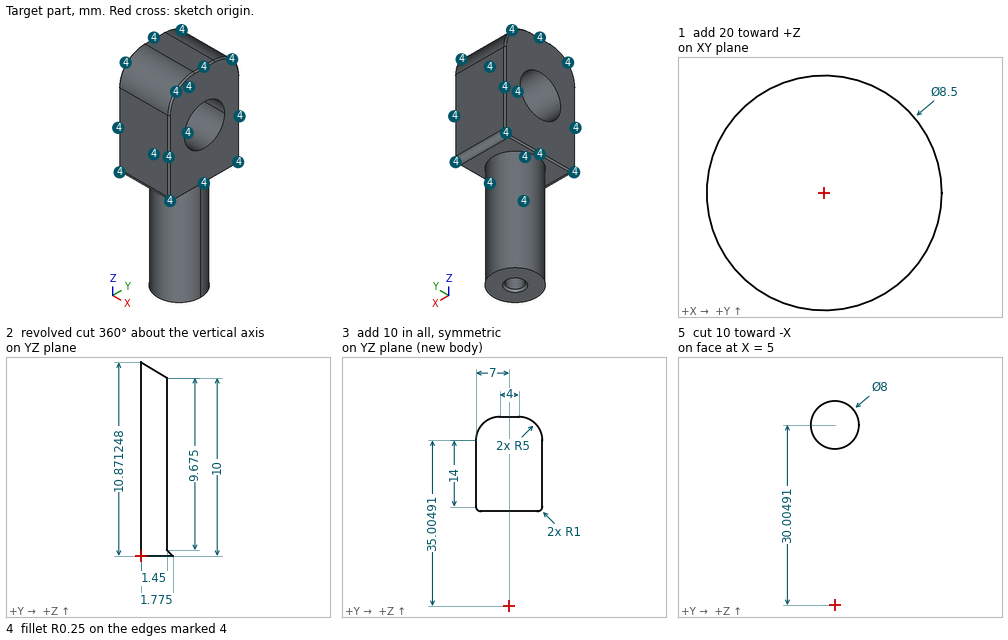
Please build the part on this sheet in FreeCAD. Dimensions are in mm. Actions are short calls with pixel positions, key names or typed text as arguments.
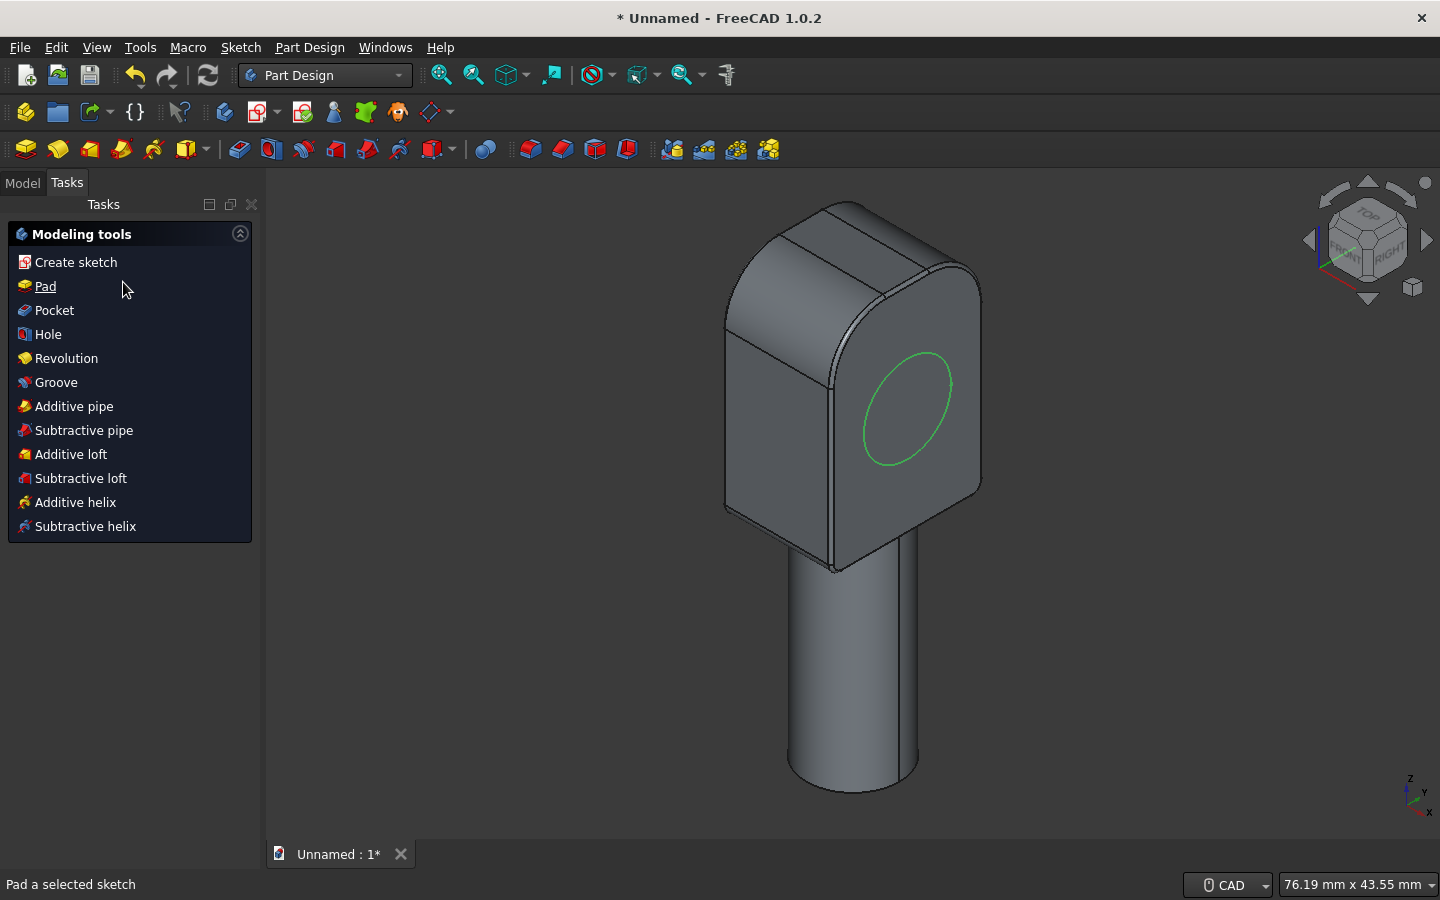
click(240, 150)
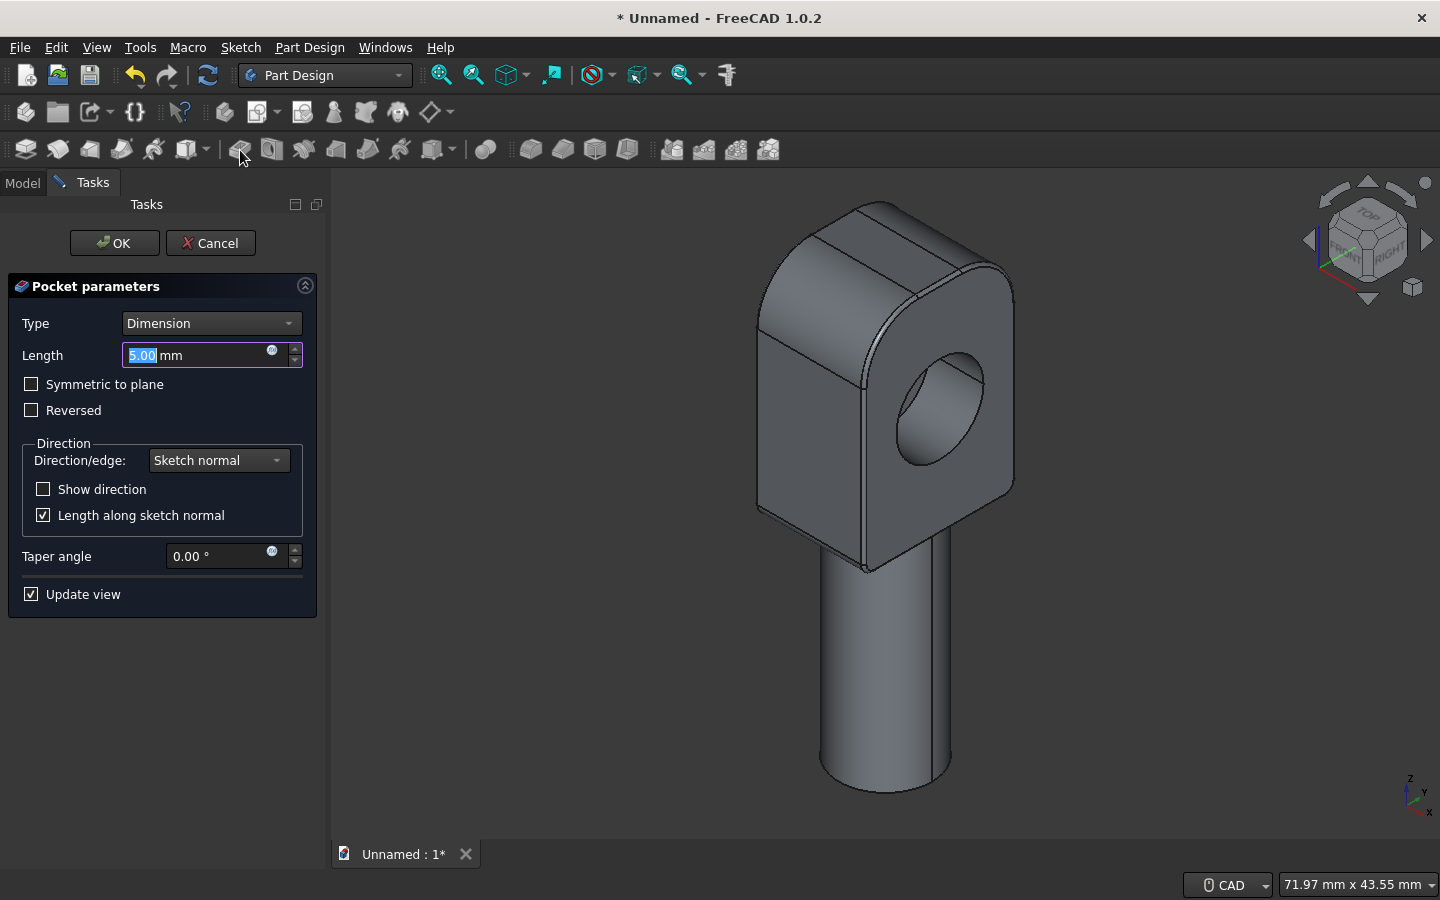
text(10)
key(Tab)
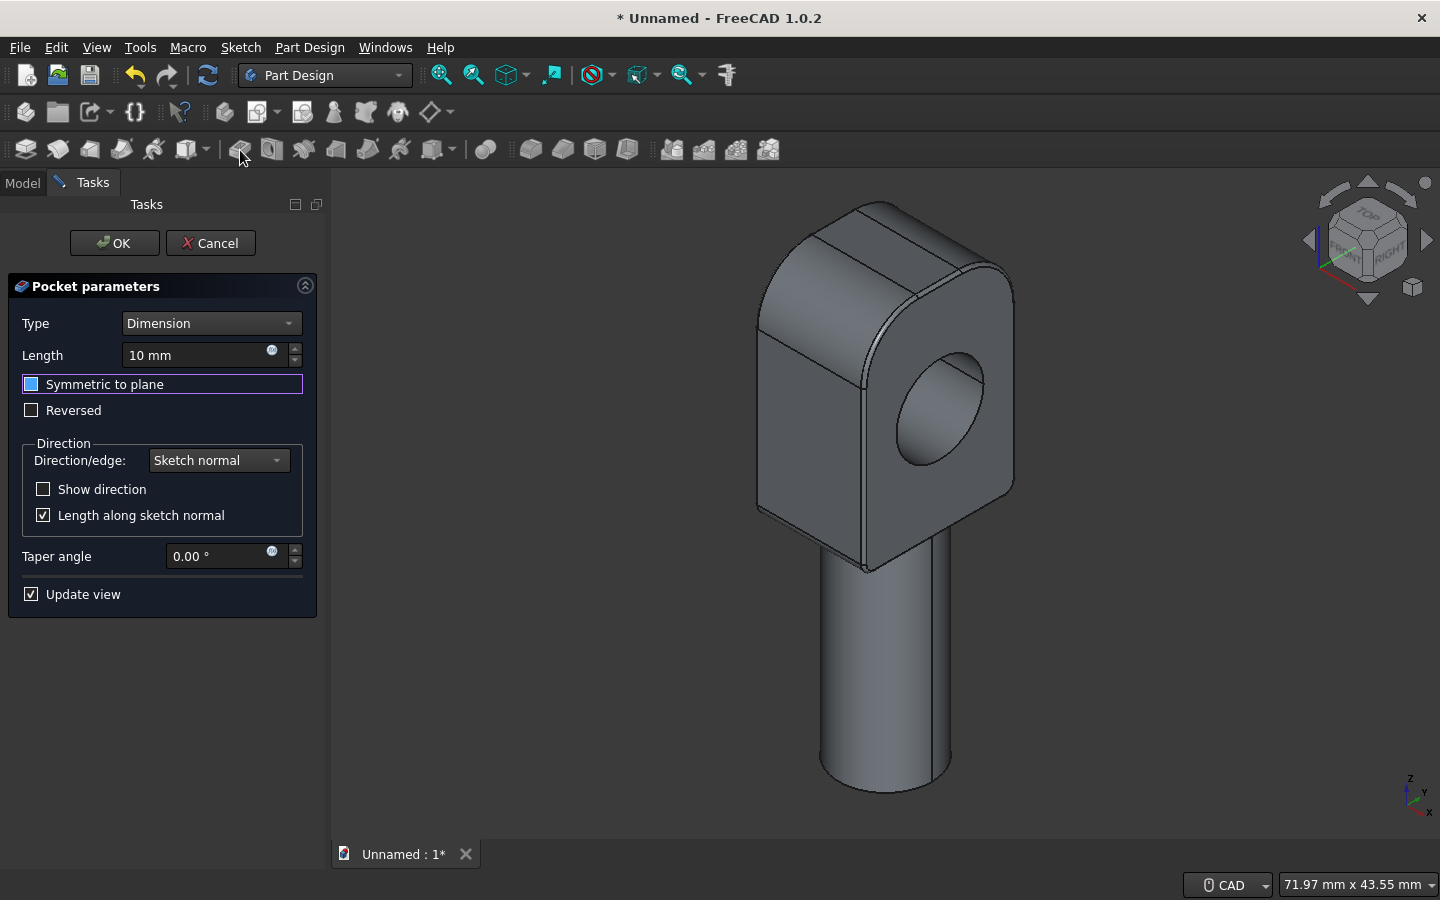
click(115, 243)